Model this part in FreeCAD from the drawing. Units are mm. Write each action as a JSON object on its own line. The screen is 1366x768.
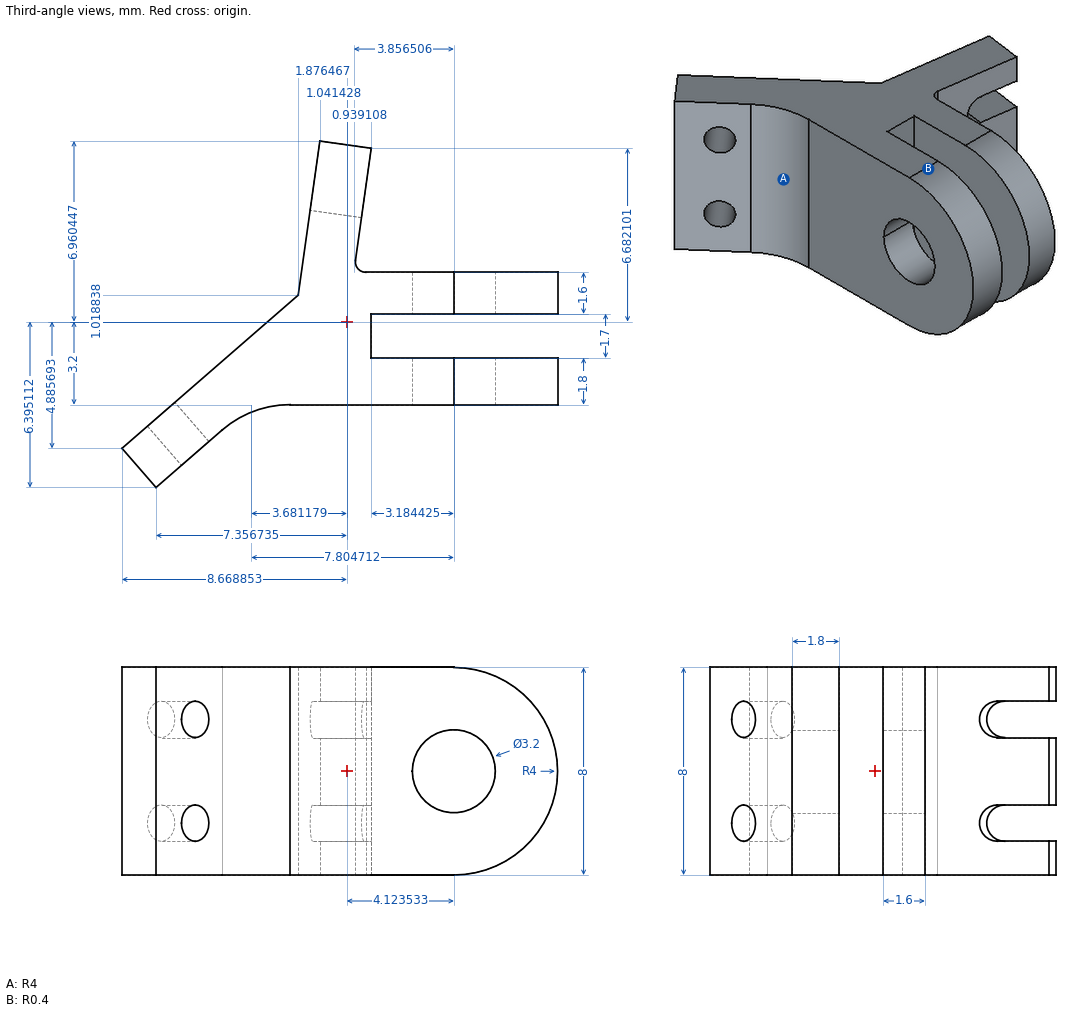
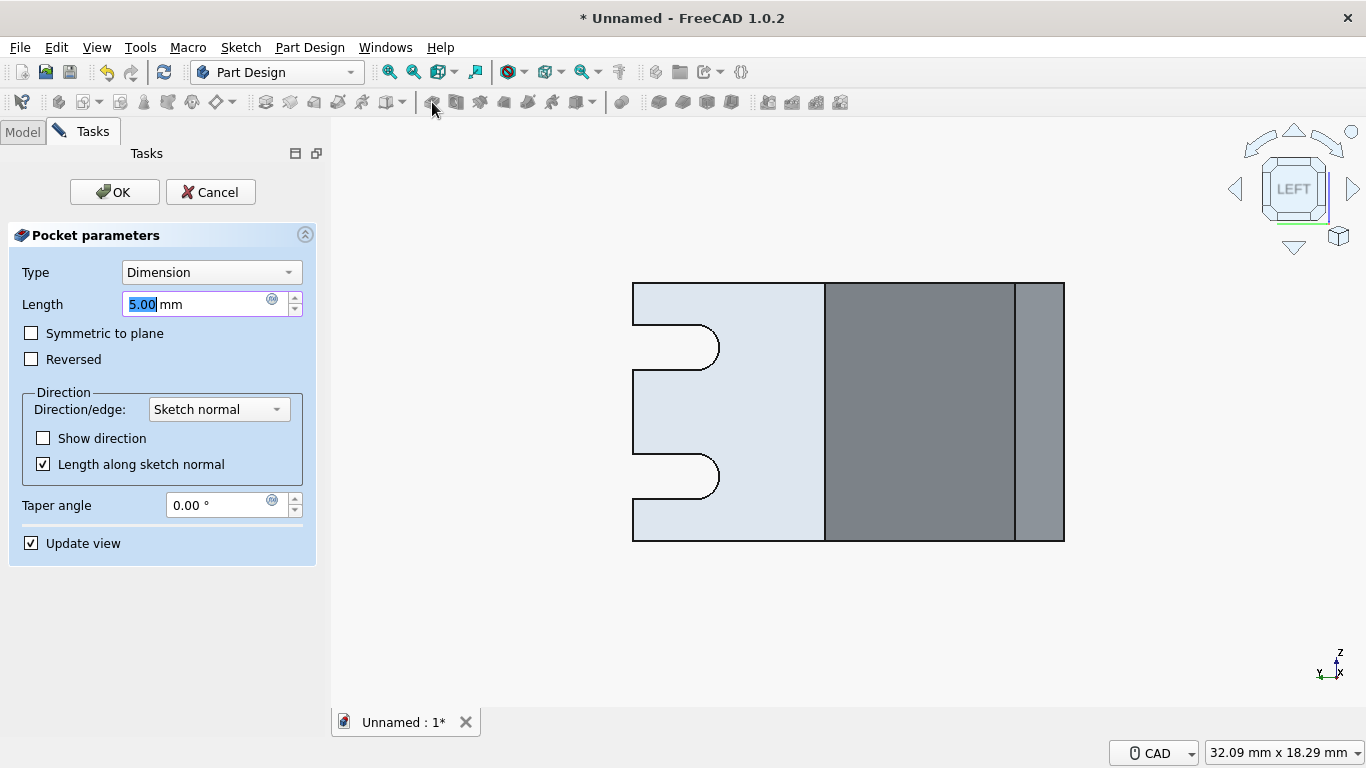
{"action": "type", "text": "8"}
{"action": "key", "text": "Tab"}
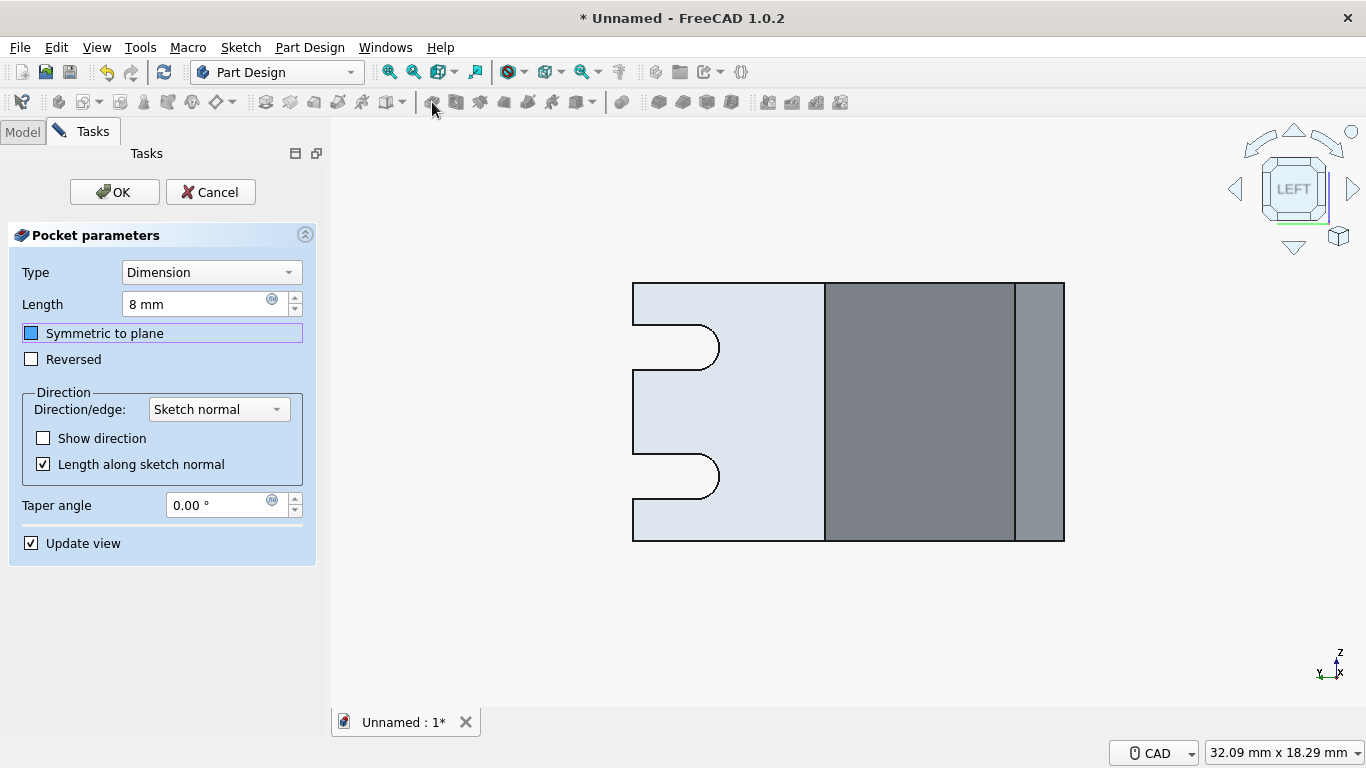
{"action": "left_click", "coordinate": [115, 192]}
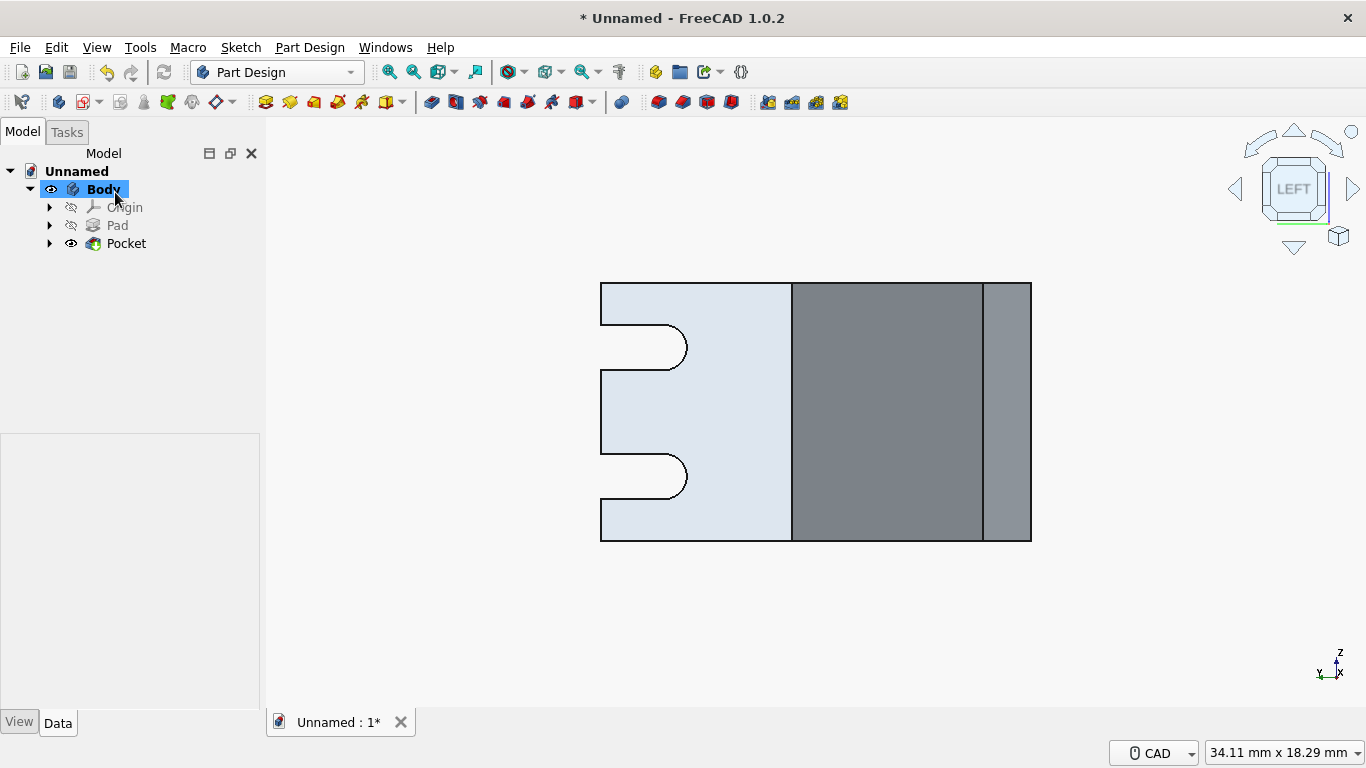
{"action": "left_click", "coordinate": [390, 72]}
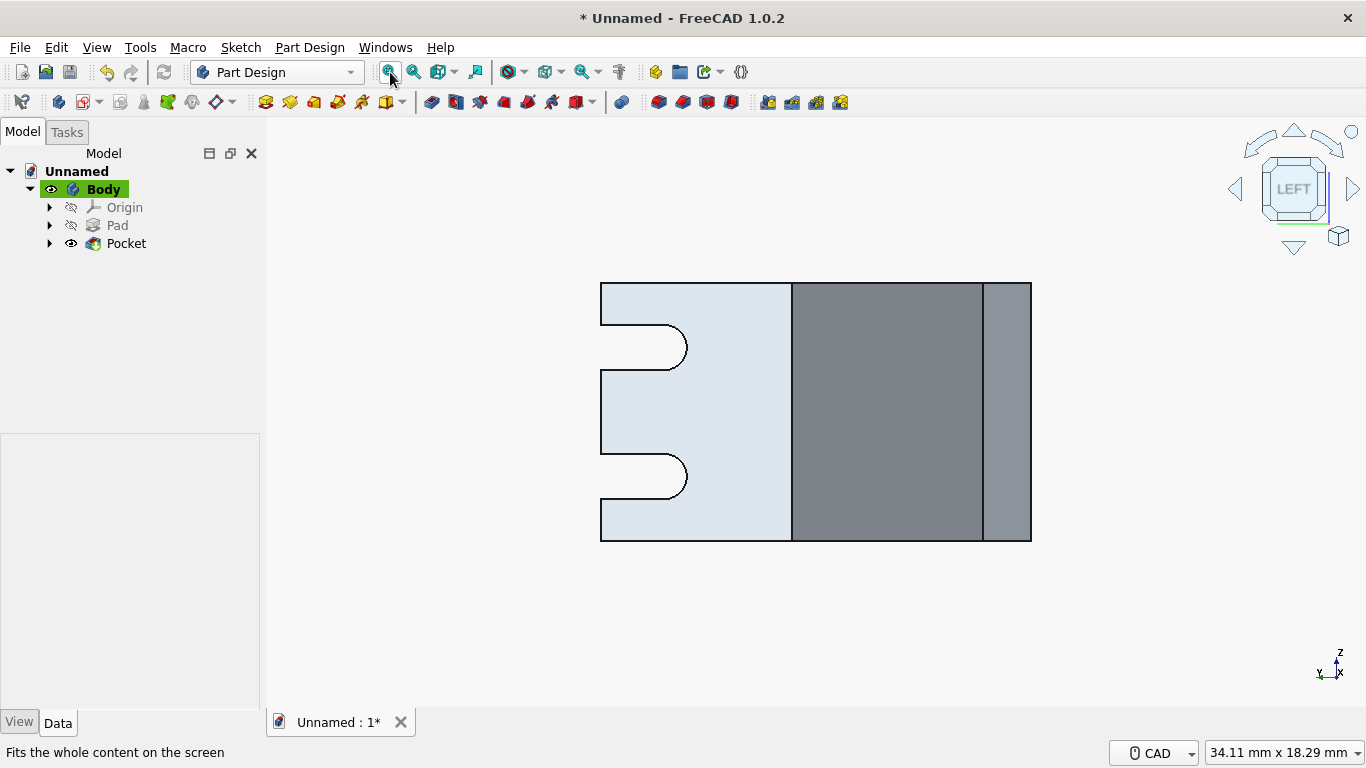
{"action": "left_click", "coordinate": [887, 411]}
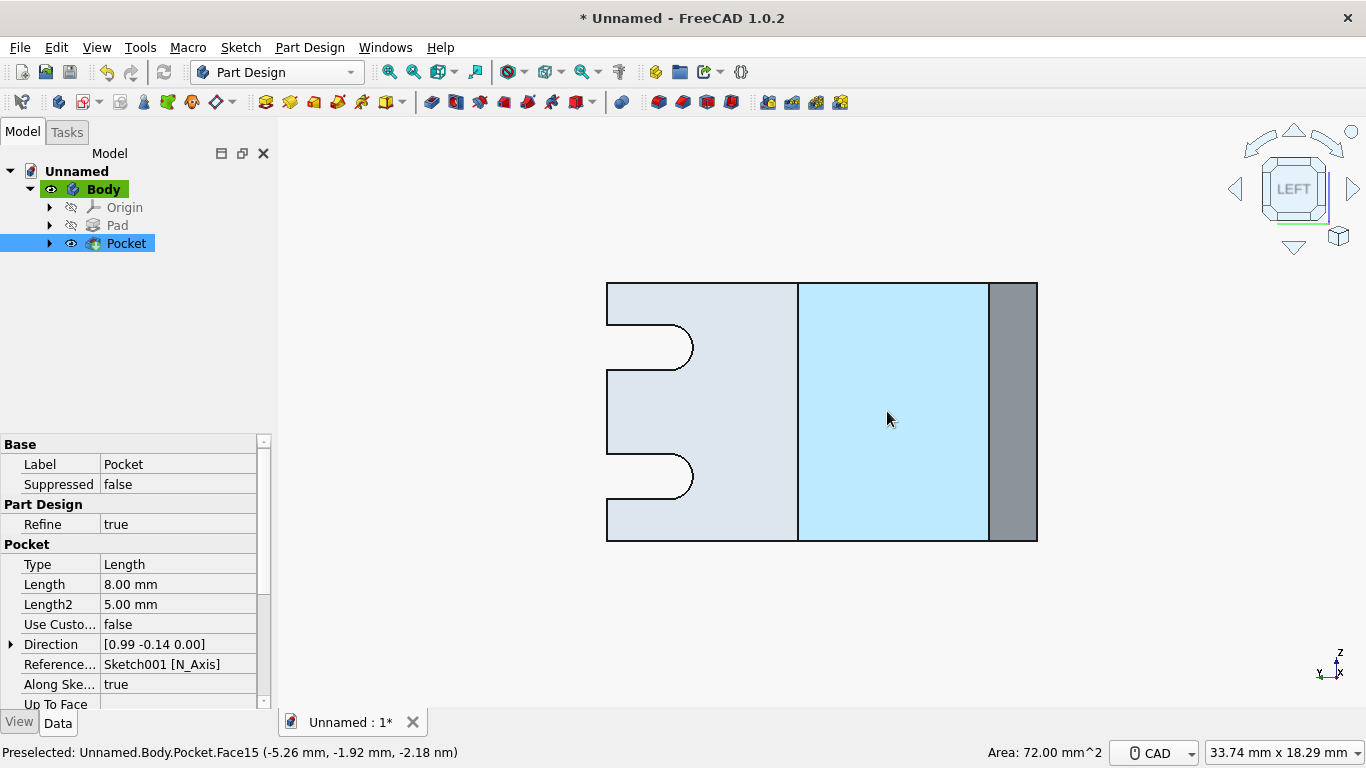
{"action": "left_click", "coordinate": [84, 102]}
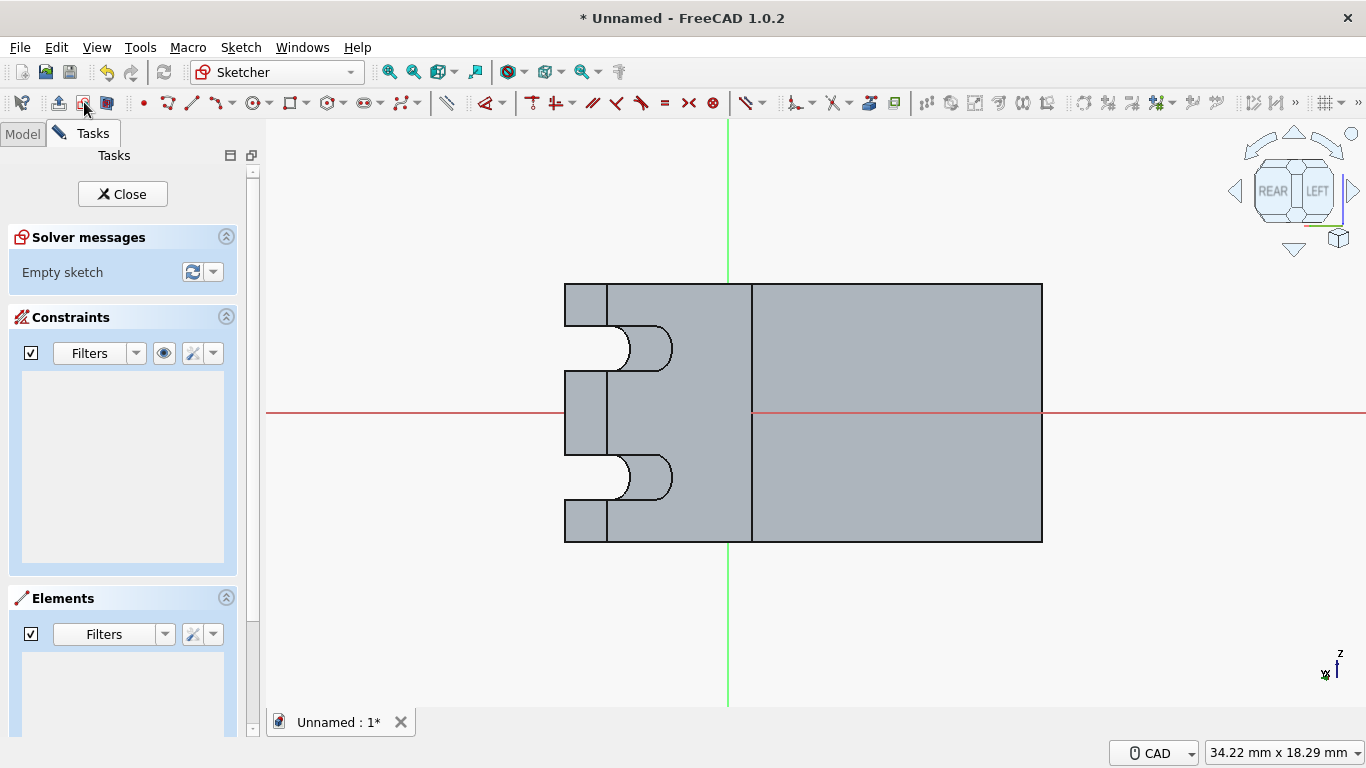
{"action": "left_click", "coordinate": [108, 104]}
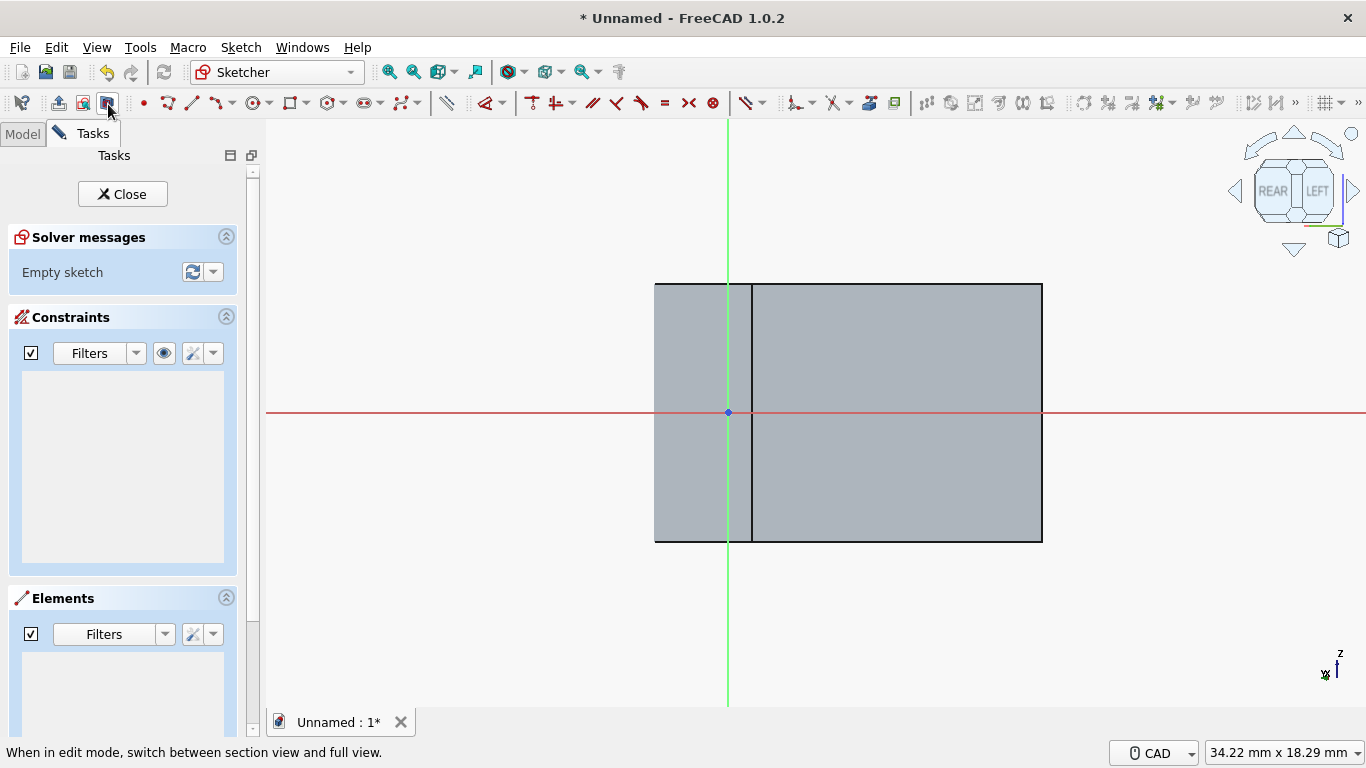
{"action": "scroll", "coordinate": [959, 413], "scroll_direction": "up", "scroll_amount": 4}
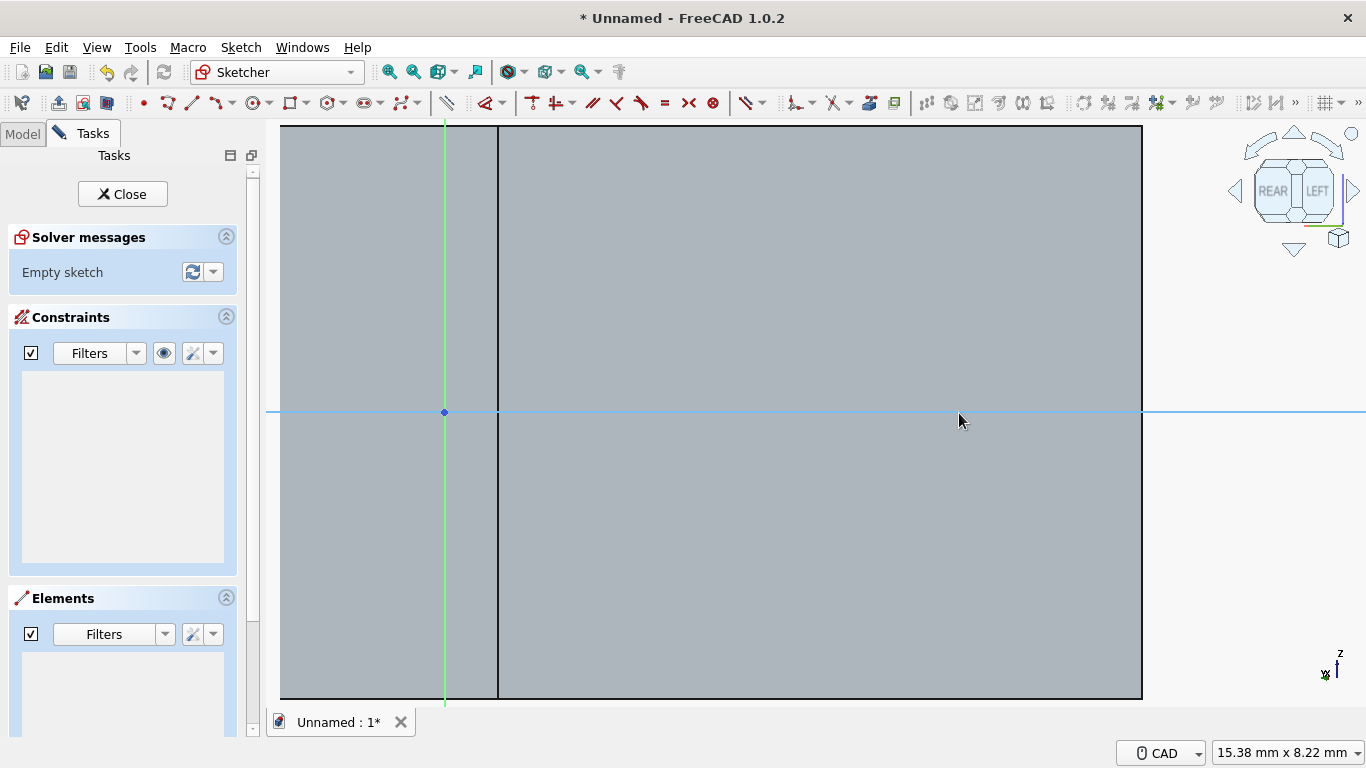
{"action": "left_click", "coordinate": [254, 104]}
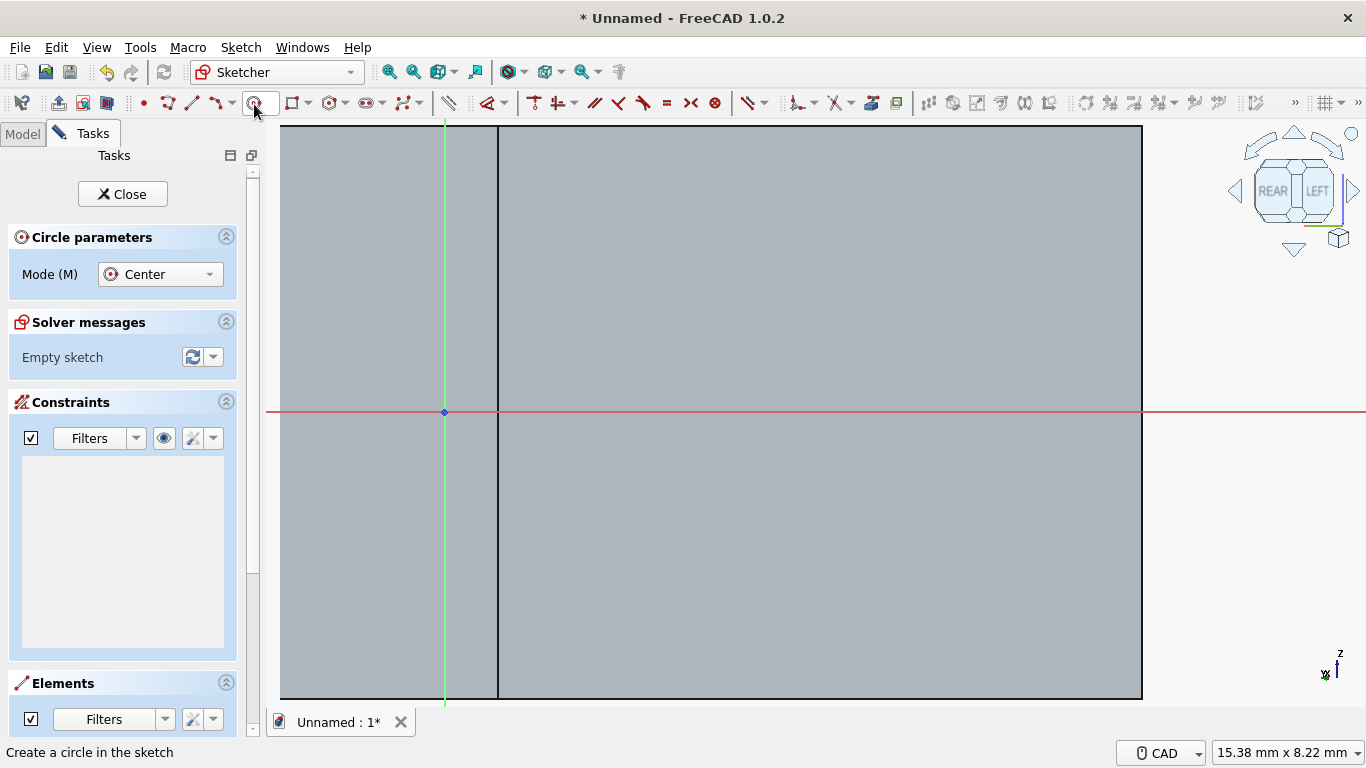
{"action": "left_click", "coordinate": [999, 269]}
{"action": "mouse_move", "coordinate": [1034, 234]}